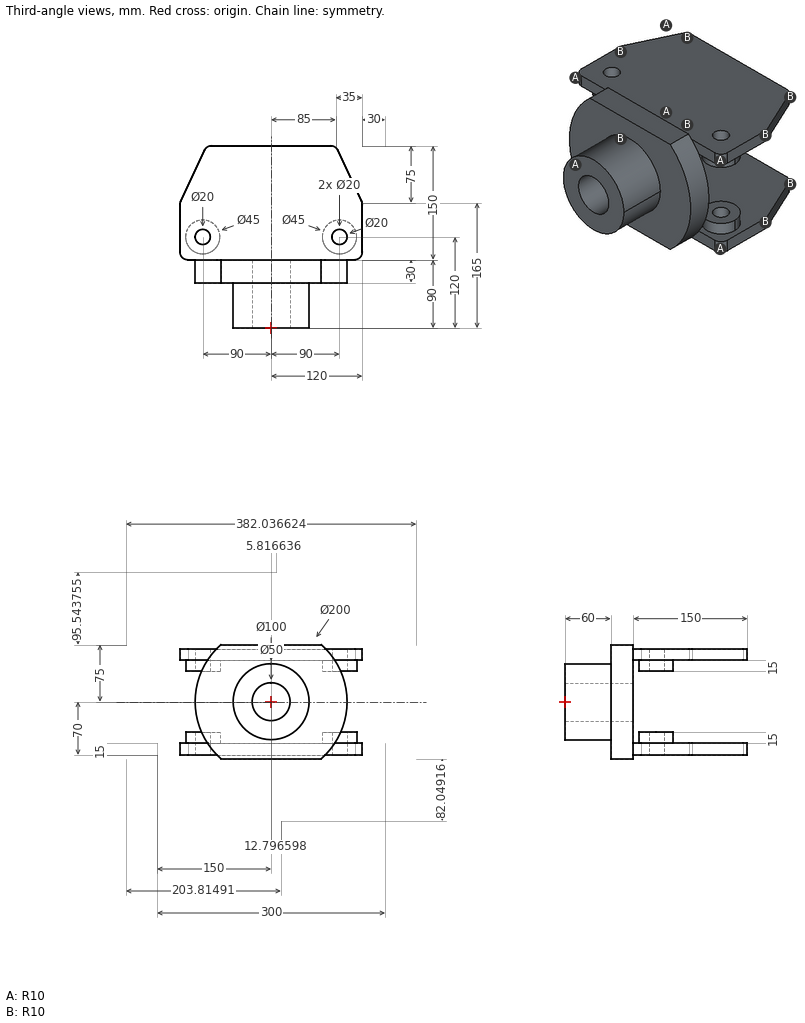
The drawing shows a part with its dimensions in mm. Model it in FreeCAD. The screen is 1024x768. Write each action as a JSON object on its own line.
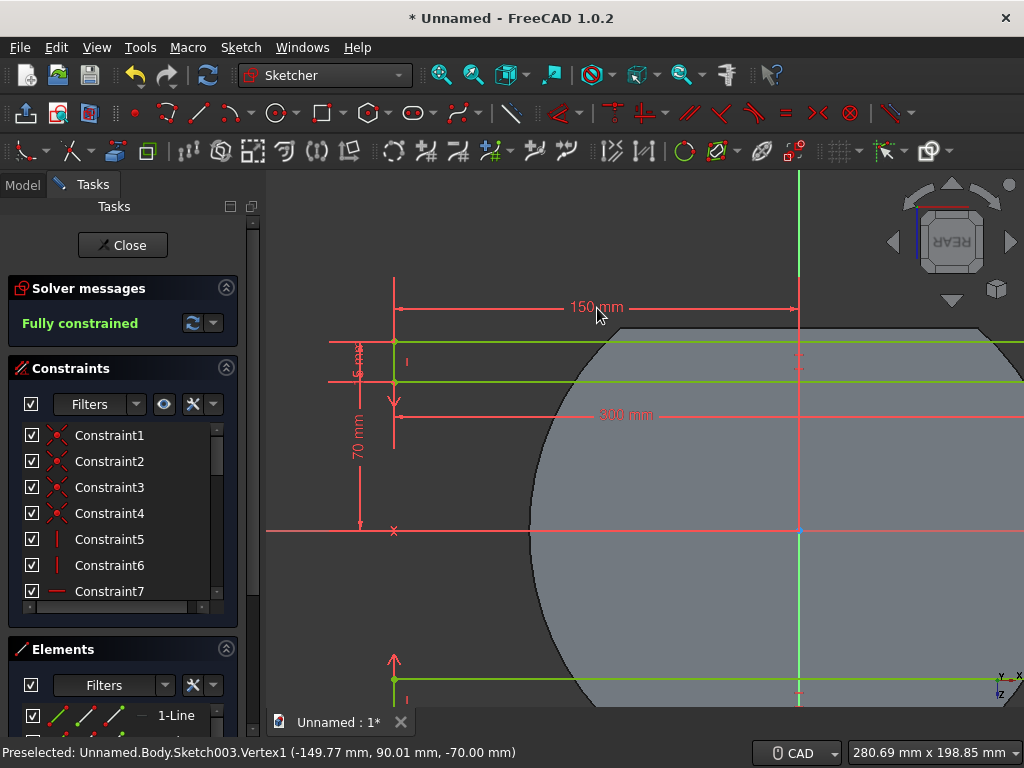
{"action": "left_click", "coordinate": [123, 245]}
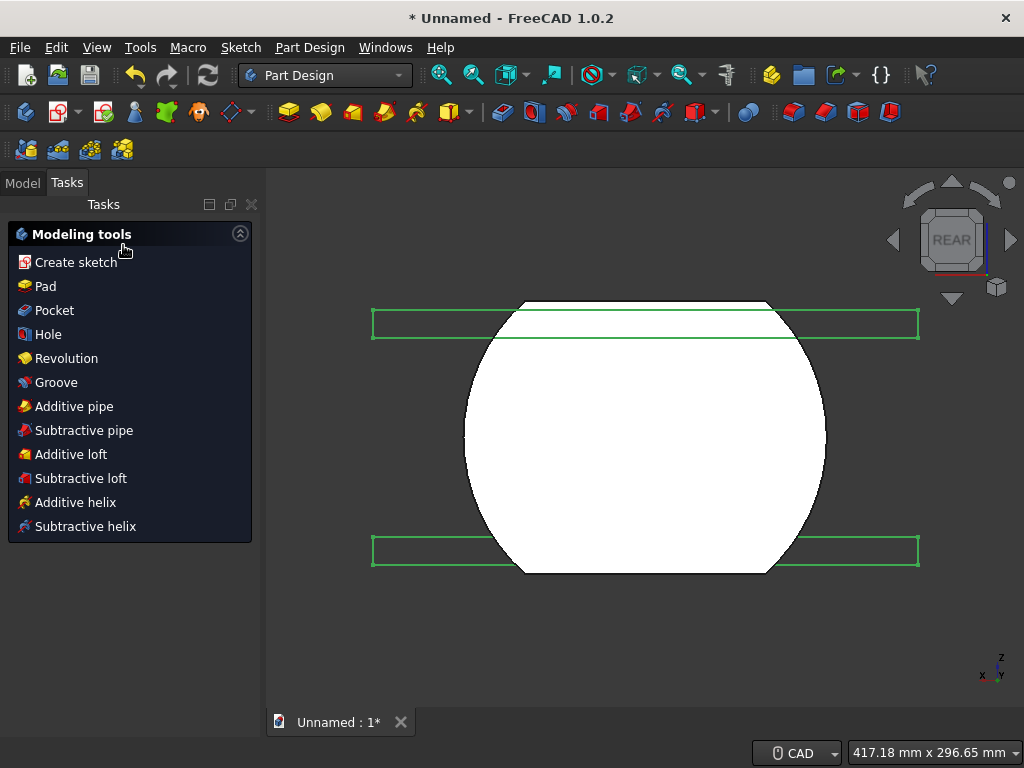
{"action": "left_click", "coordinate": [290, 112]}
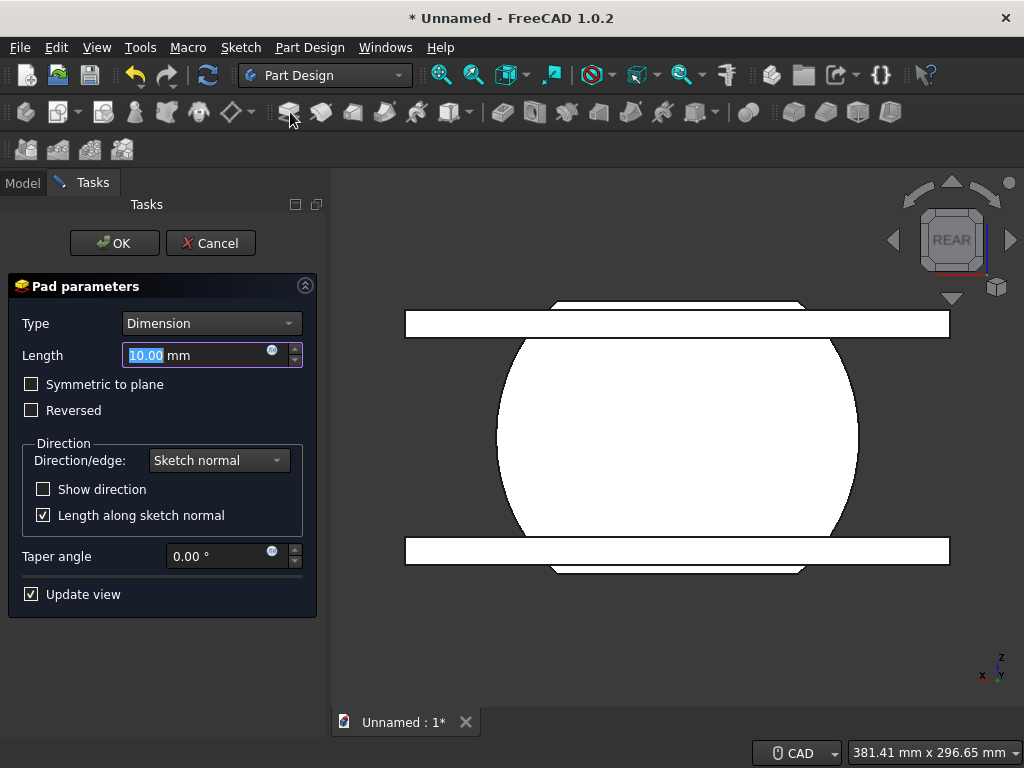
{"action": "type", "text": "150"}
{"action": "key", "text": "Tab"}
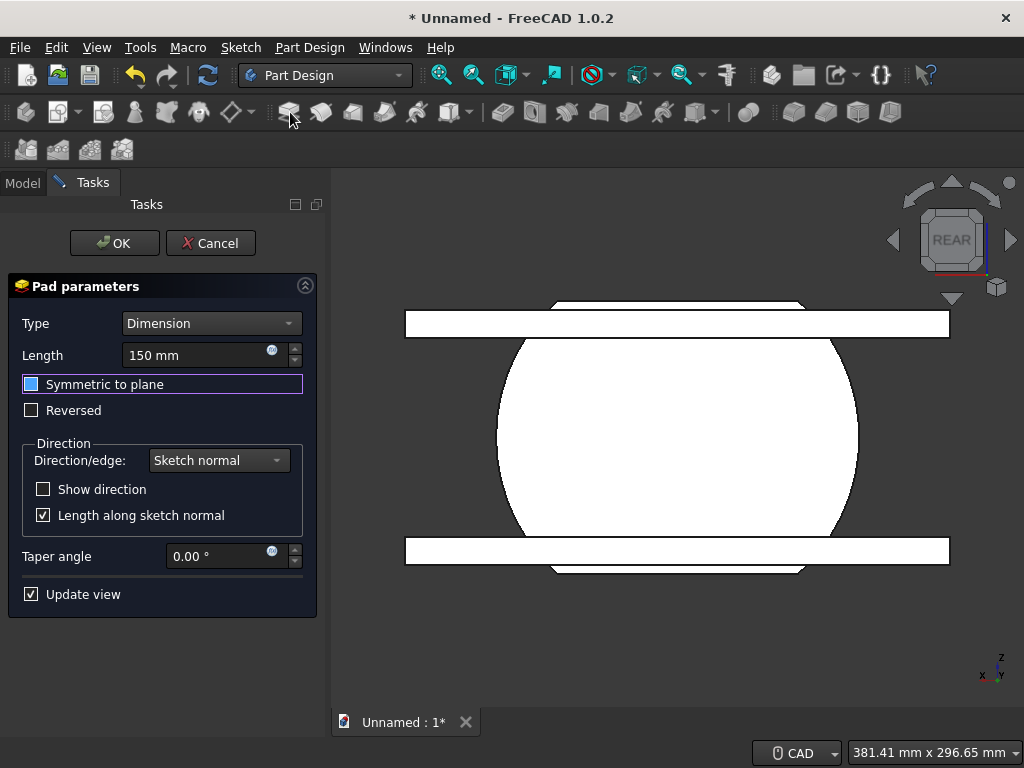
{"action": "left_click", "coordinate": [115, 243]}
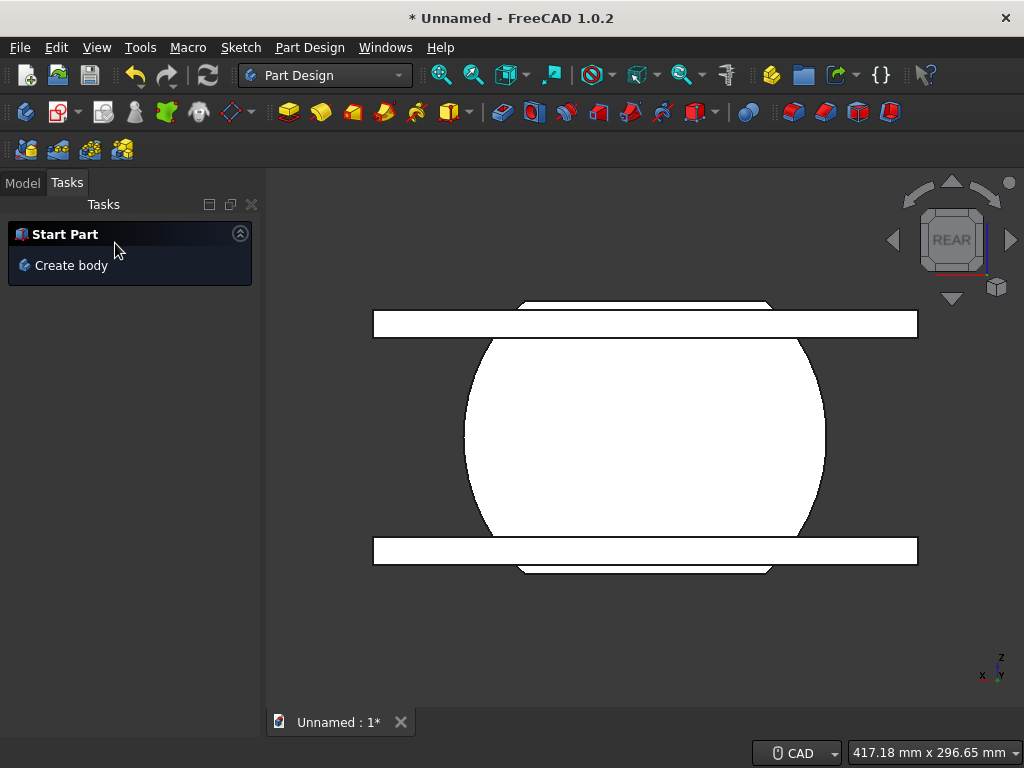
{"action": "key", "text": "5"}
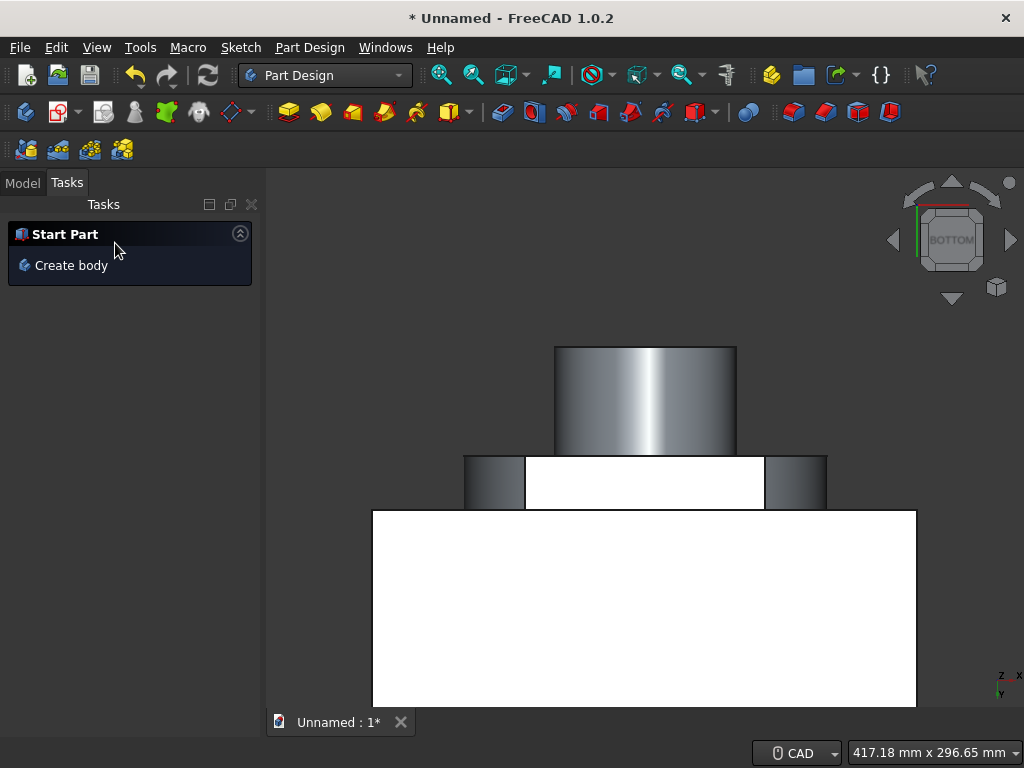
{"action": "left_click", "coordinate": [442, 76]}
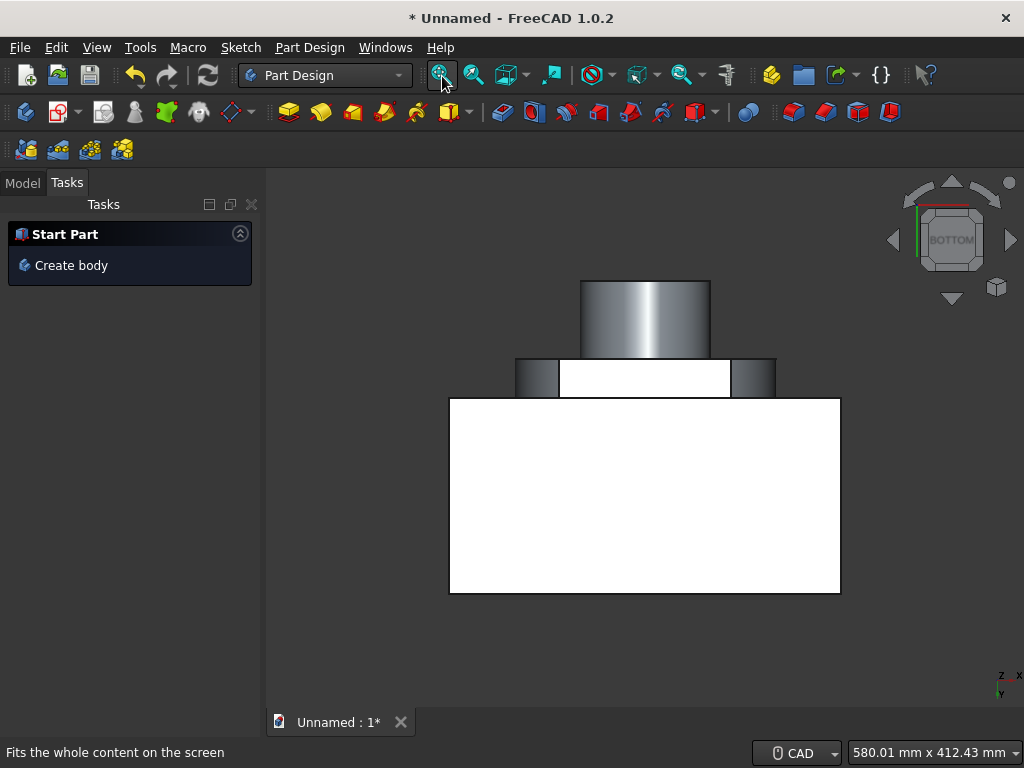
{"action": "left_click", "coordinate": [701, 495]}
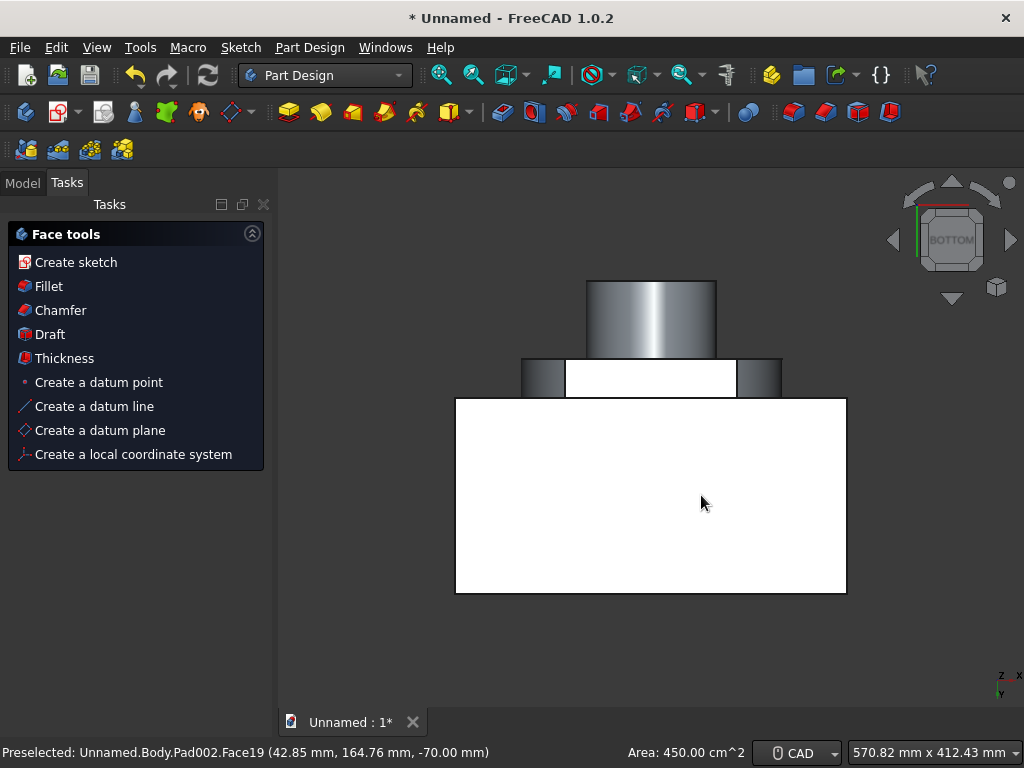
{"action": "left_click", "coordinate": [58, 112]}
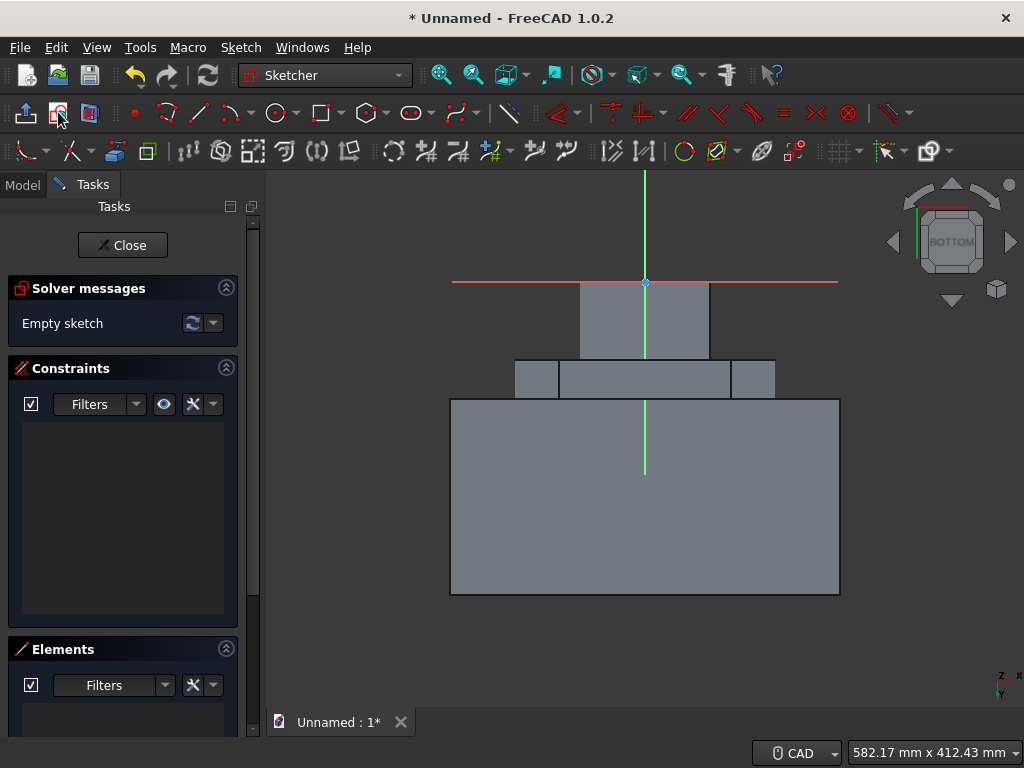
{"action": "left_click", "coordinate": [90, 114]}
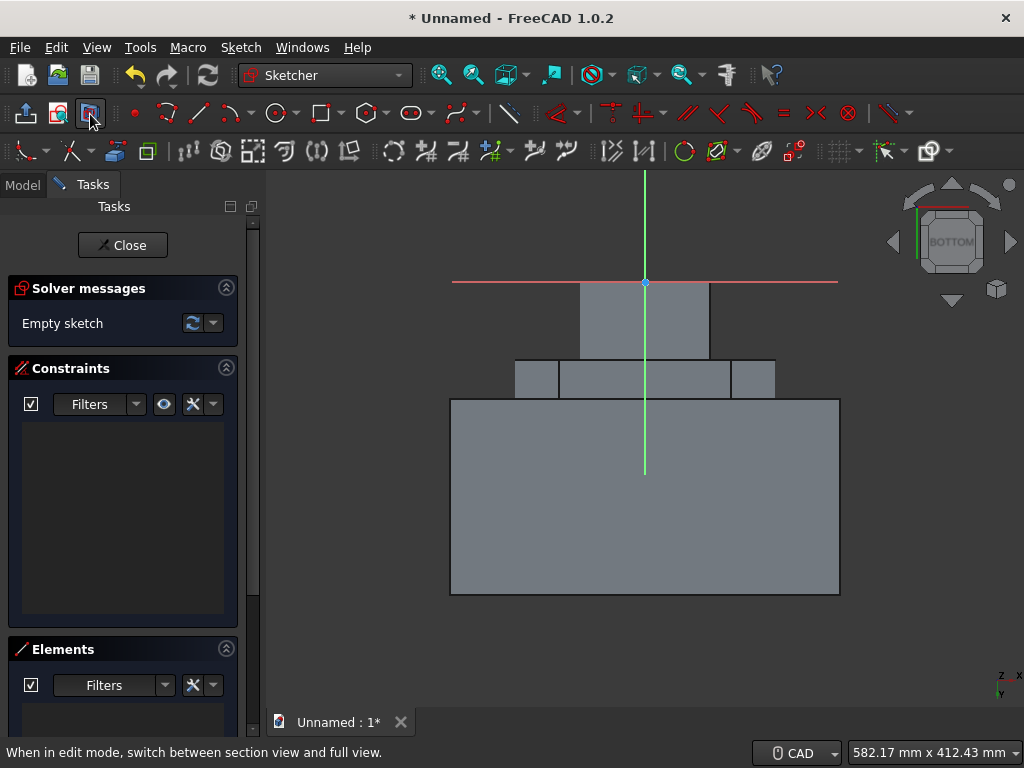
{"action": "scroll", "coordinate": [294, 439], "scroll_direction": "down", "scroll_amount": 1}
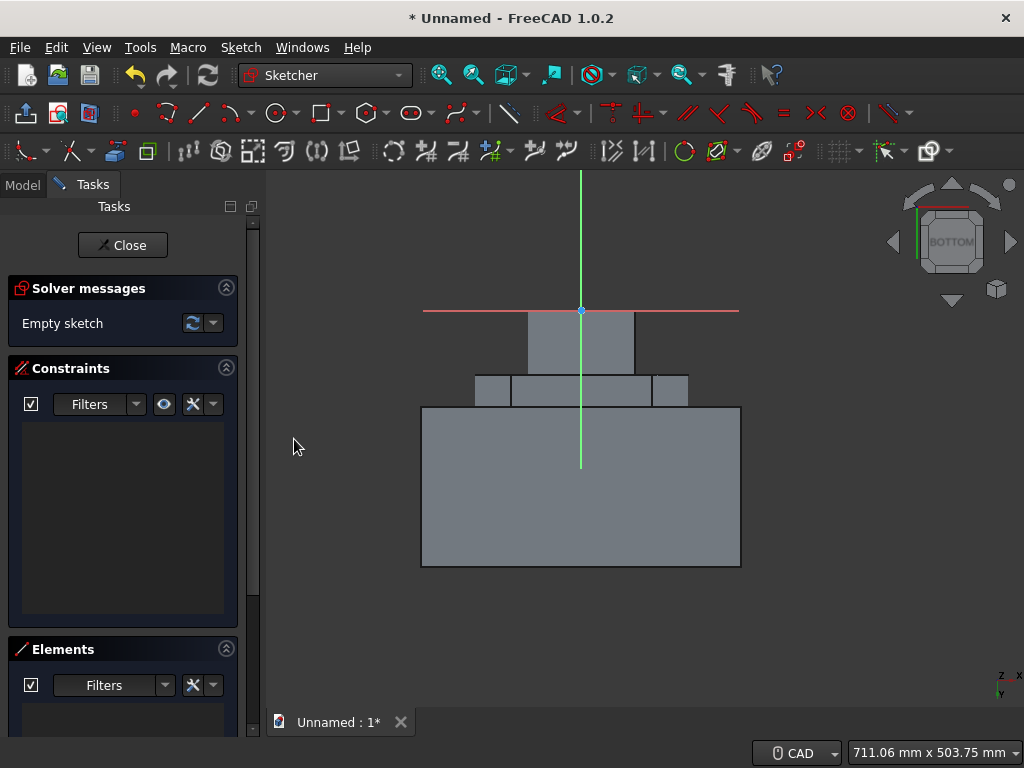
{"action": "left_click", "coordinate": [322, 114]}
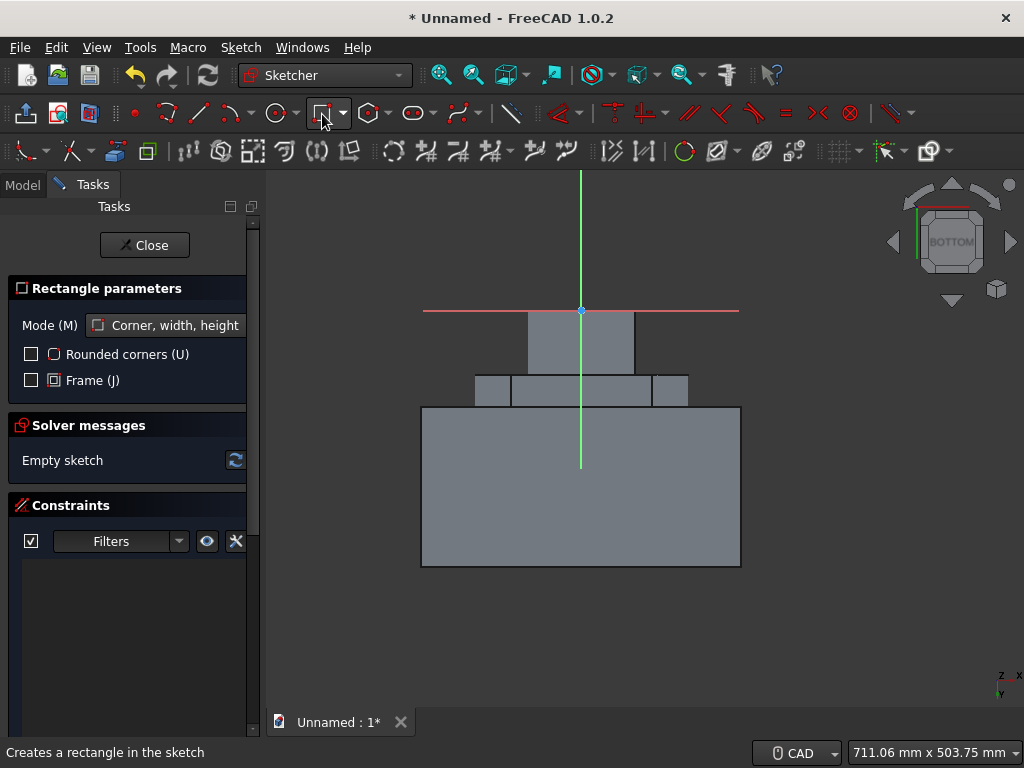
{"action": "left_click", "coordinate": [709, 407]}
{"action": "left_click", "coordinate": [741, 567]}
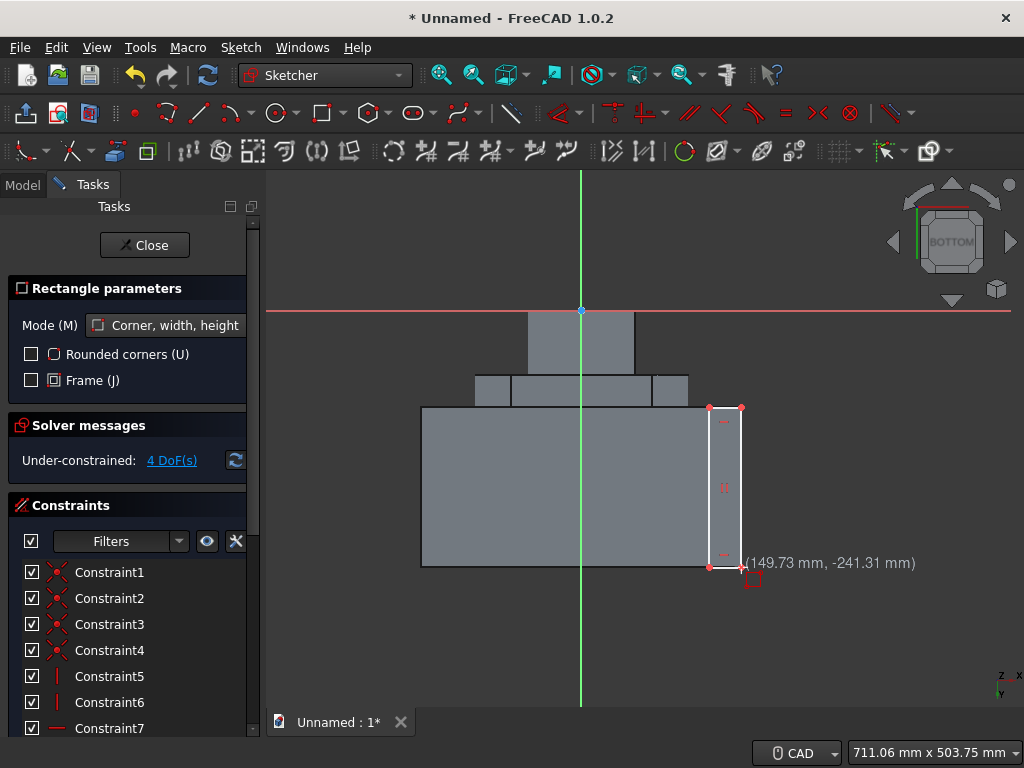
{"action": "left_click", "coordinate": [421, 407]}
{"action": "left_click", "coordinate": [453, 567]}
{"action": "key", "text": "Escape"}